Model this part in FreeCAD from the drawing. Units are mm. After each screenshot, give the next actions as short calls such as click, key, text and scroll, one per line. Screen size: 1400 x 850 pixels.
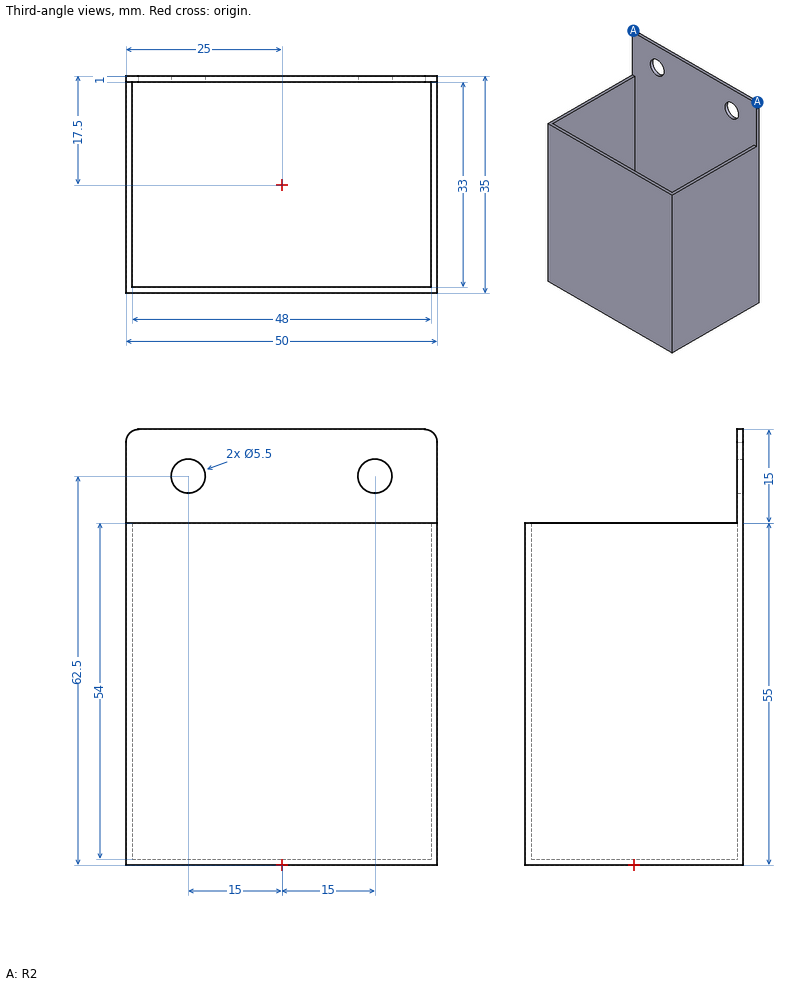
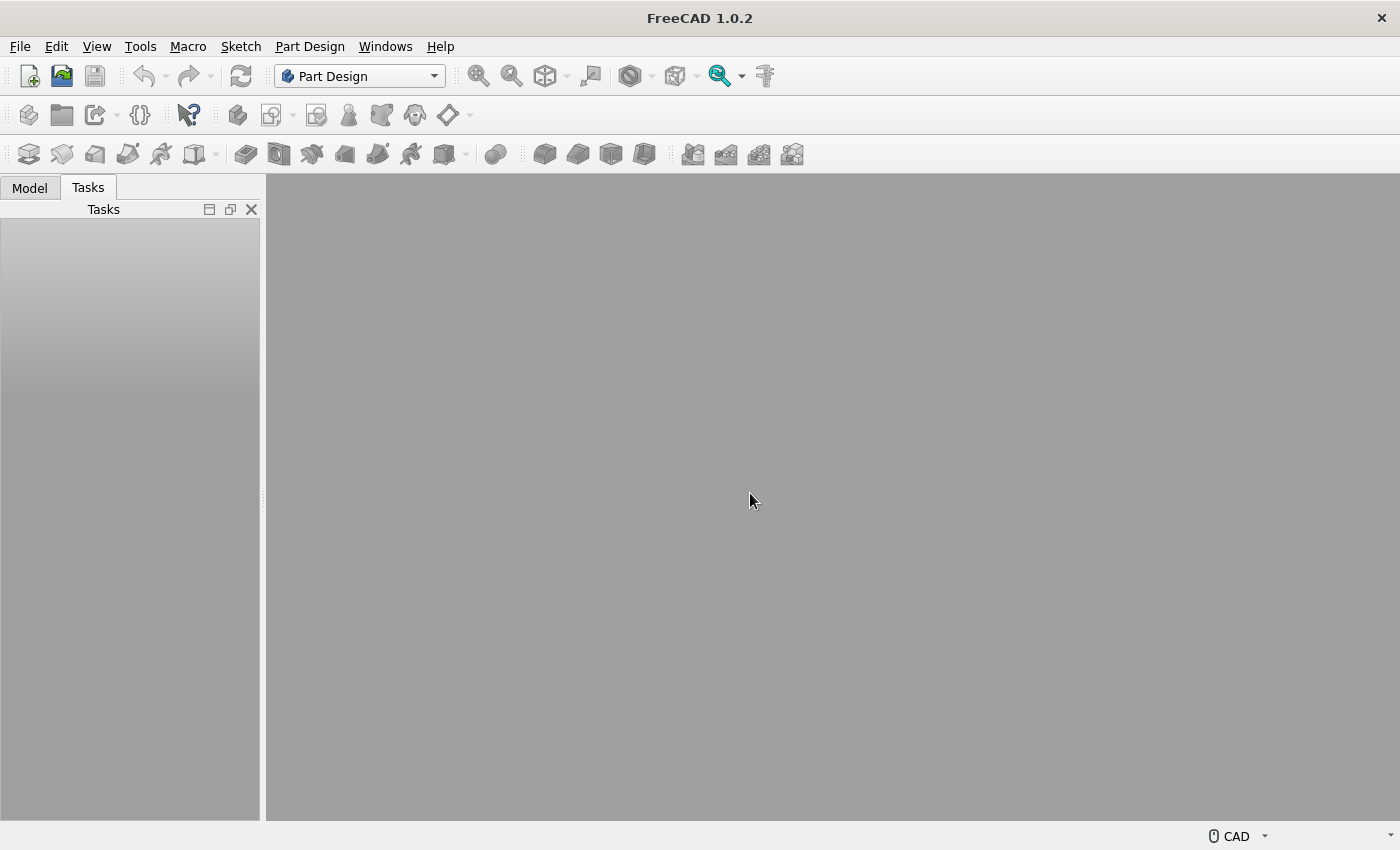
key(ctrl+n)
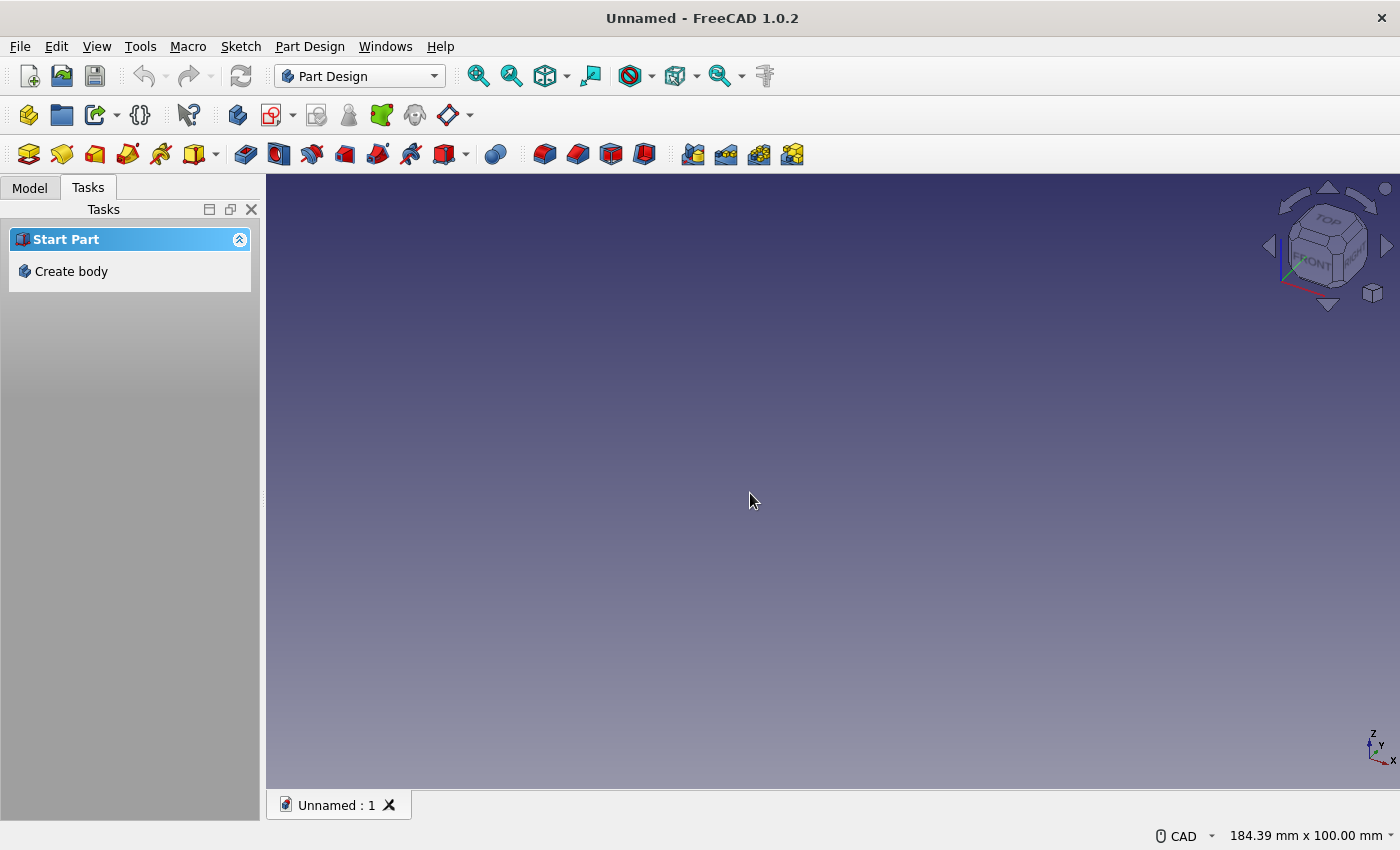
click(270, 116)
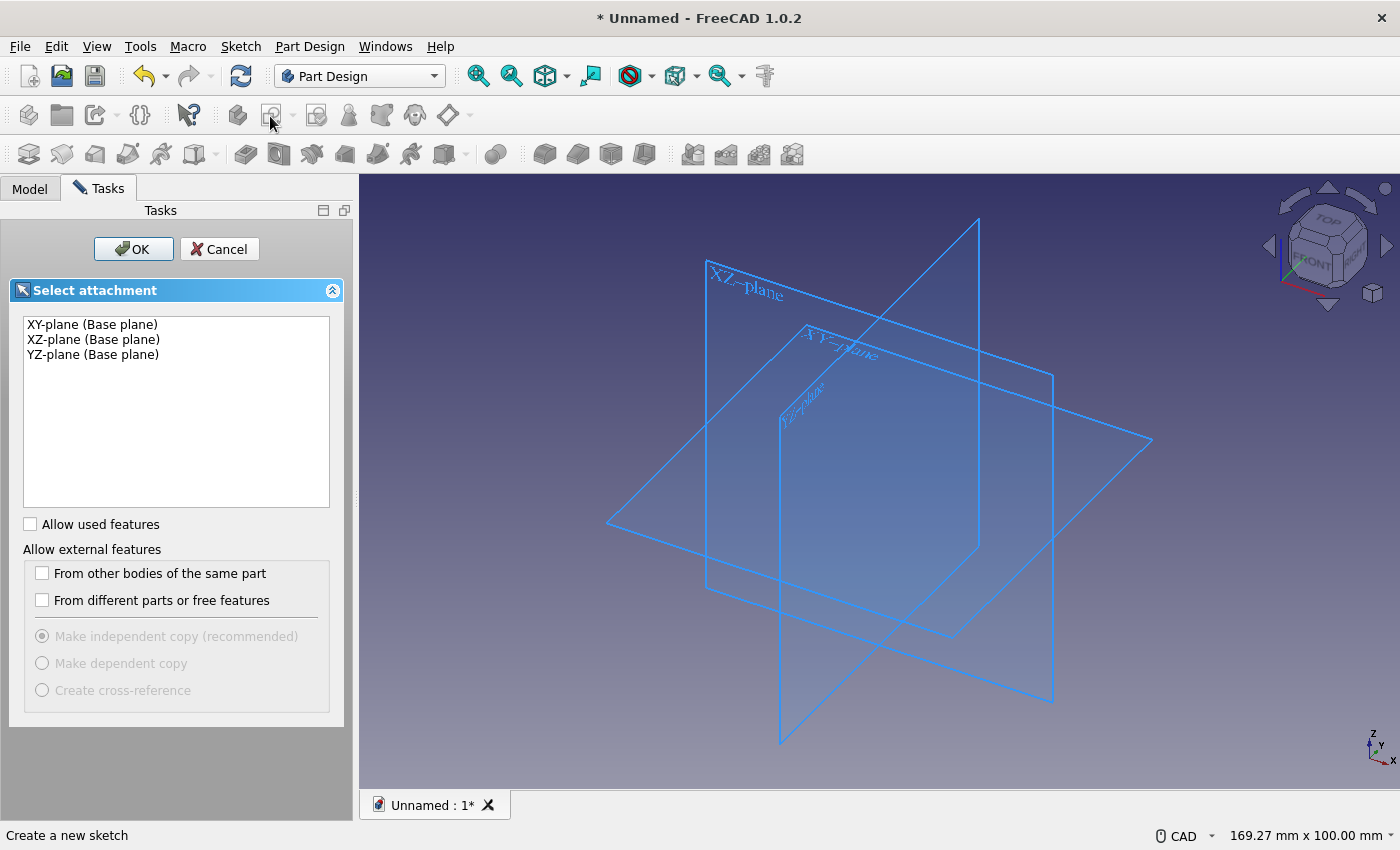
click(84, 324)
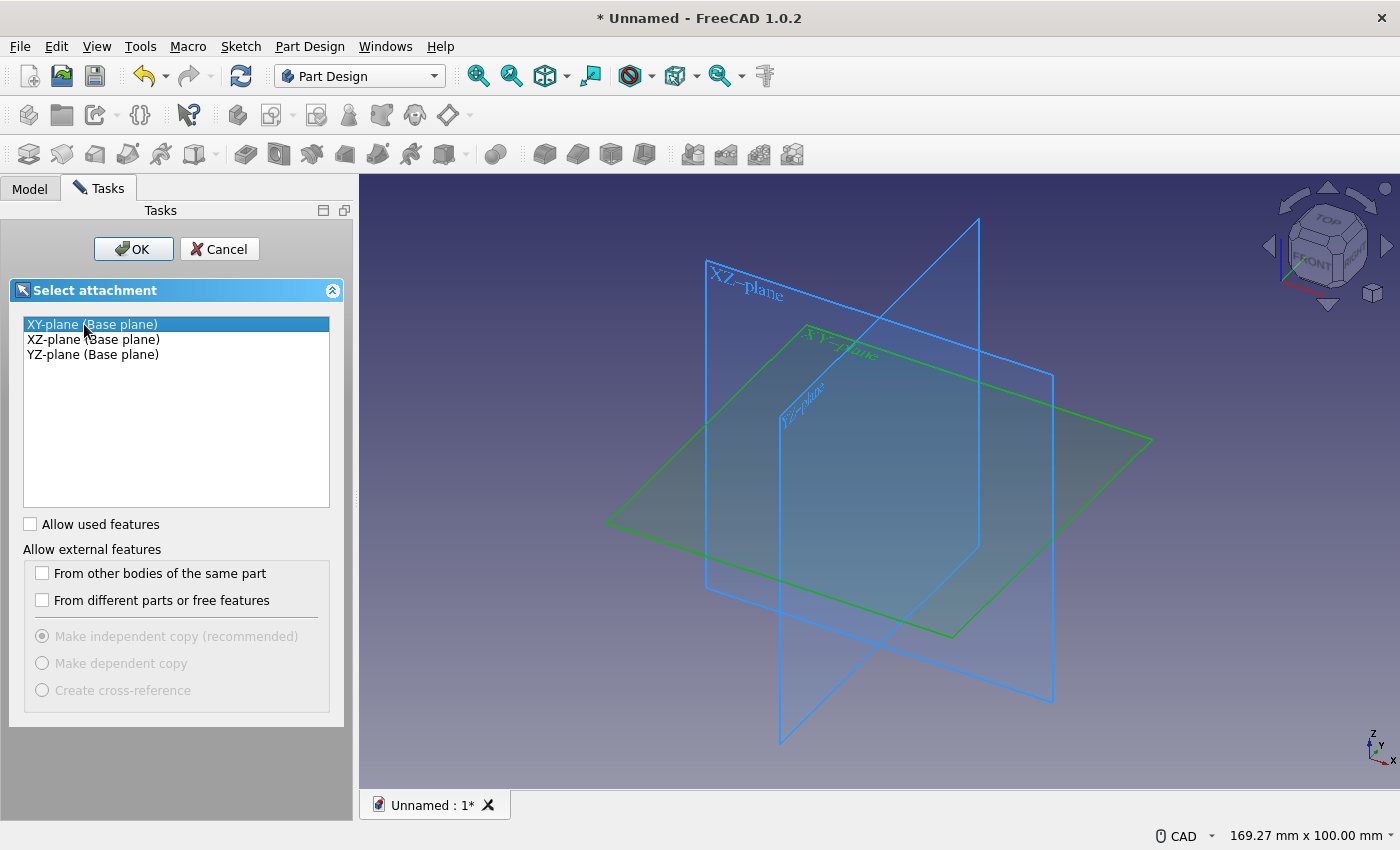
click(134, 249)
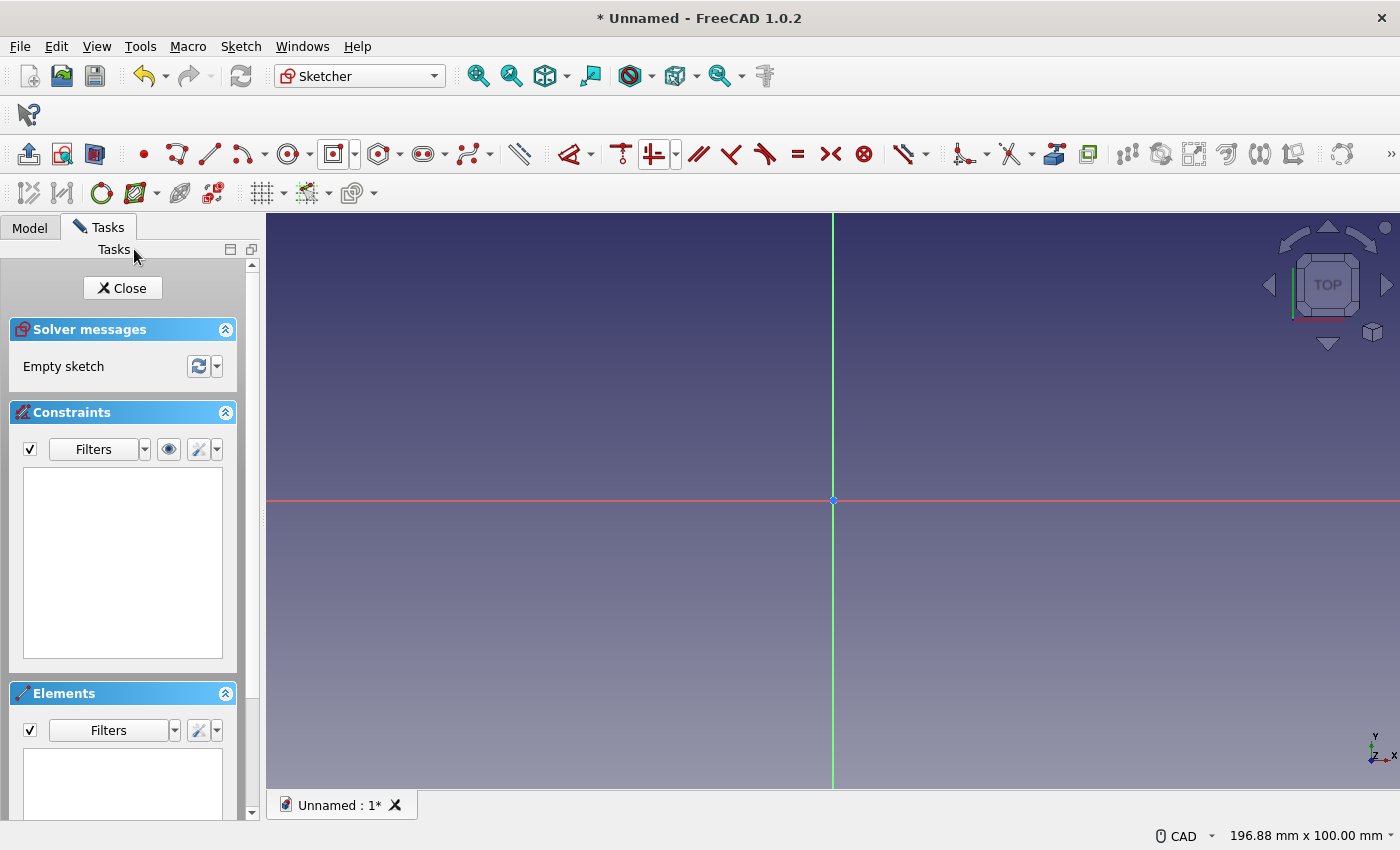
scroll(916, 501, up, 3)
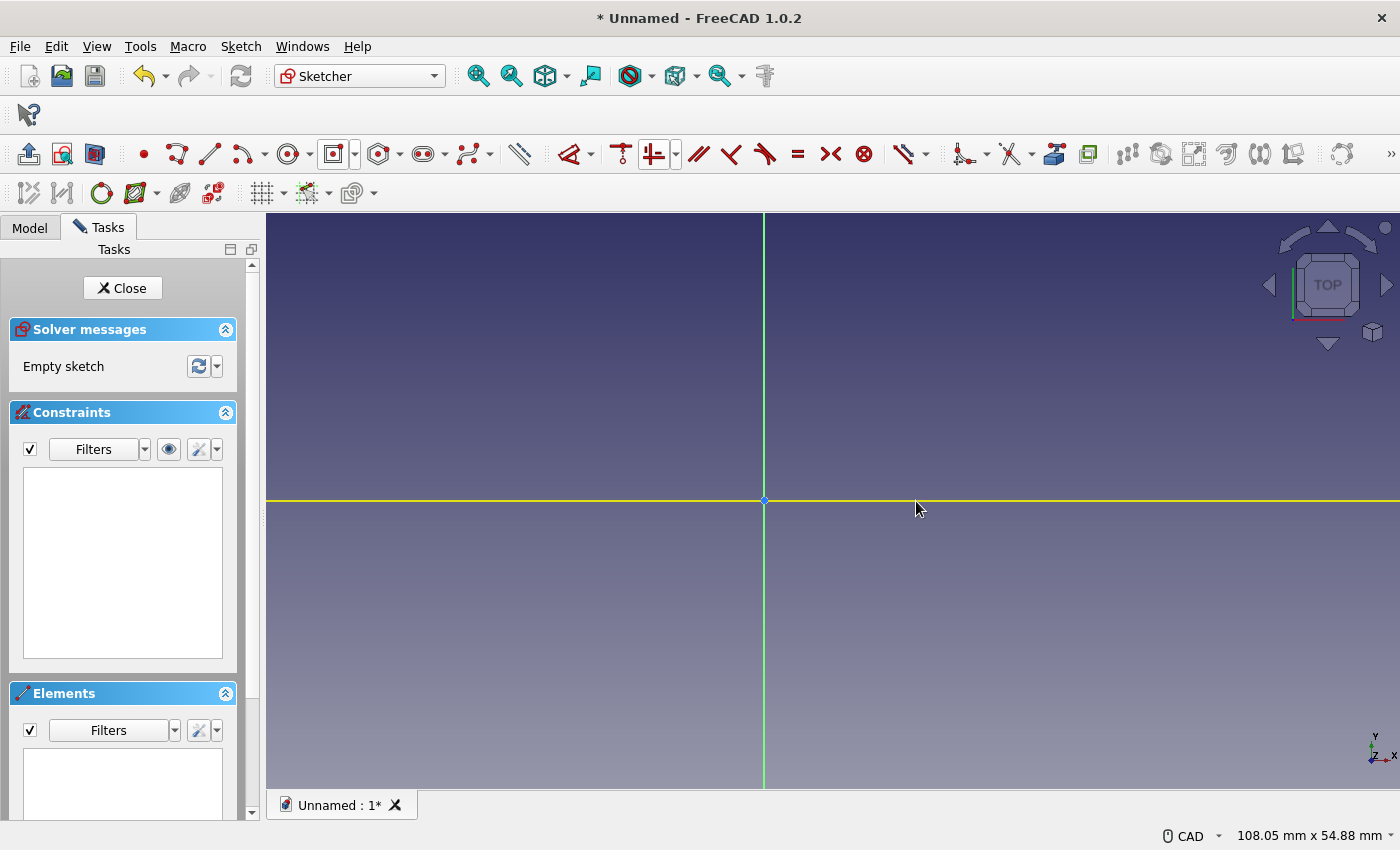
key(g)
key(v)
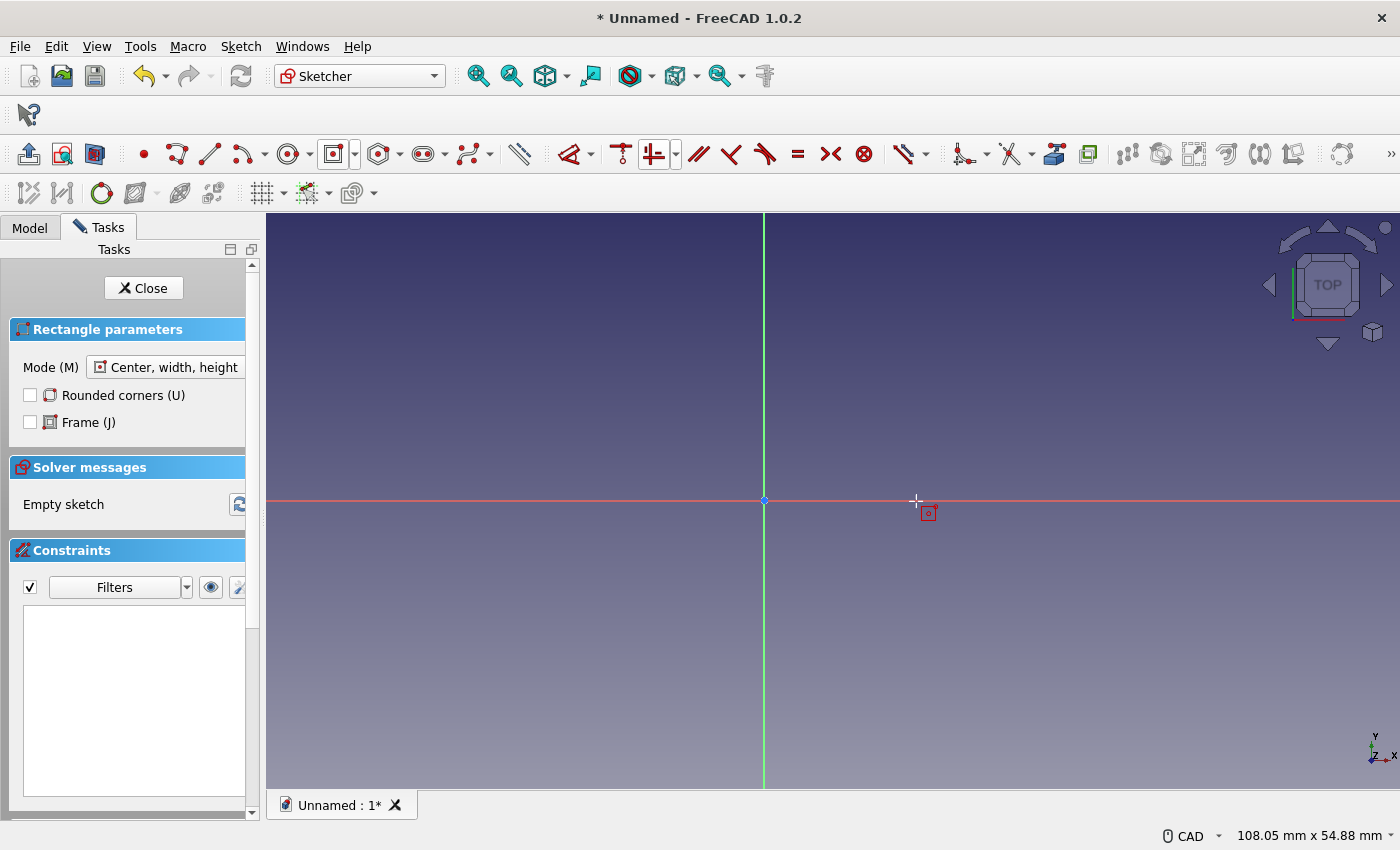
click(764, 501)
click(1027, 317)
key(Escape)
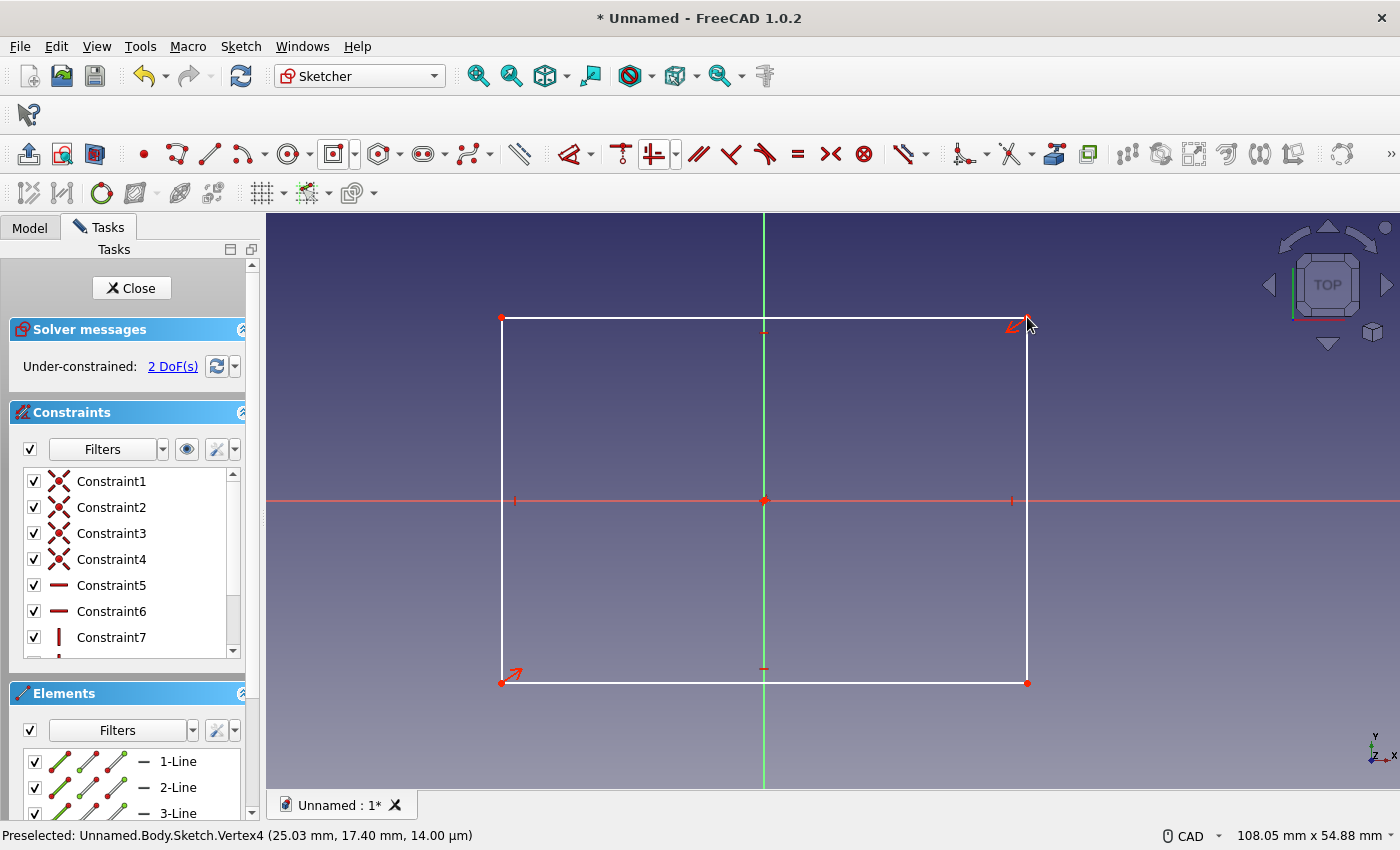
key(d)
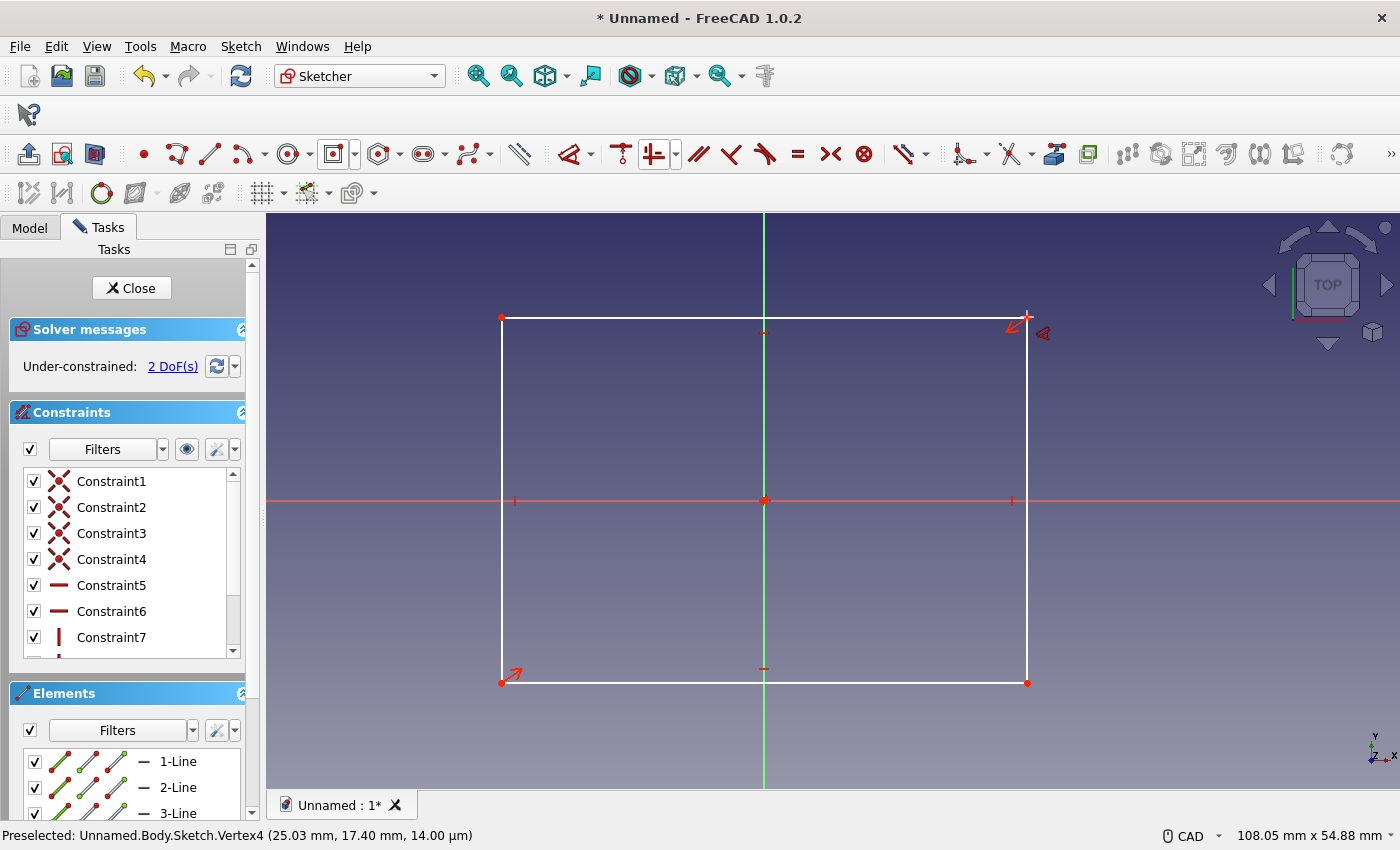
click(659, 683)
click(643, 717)